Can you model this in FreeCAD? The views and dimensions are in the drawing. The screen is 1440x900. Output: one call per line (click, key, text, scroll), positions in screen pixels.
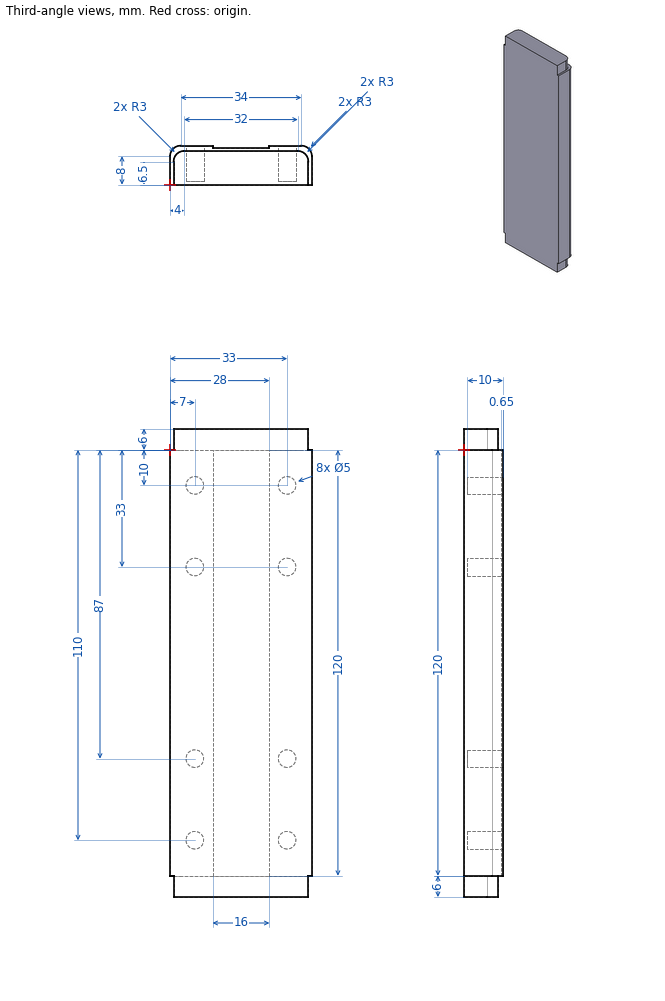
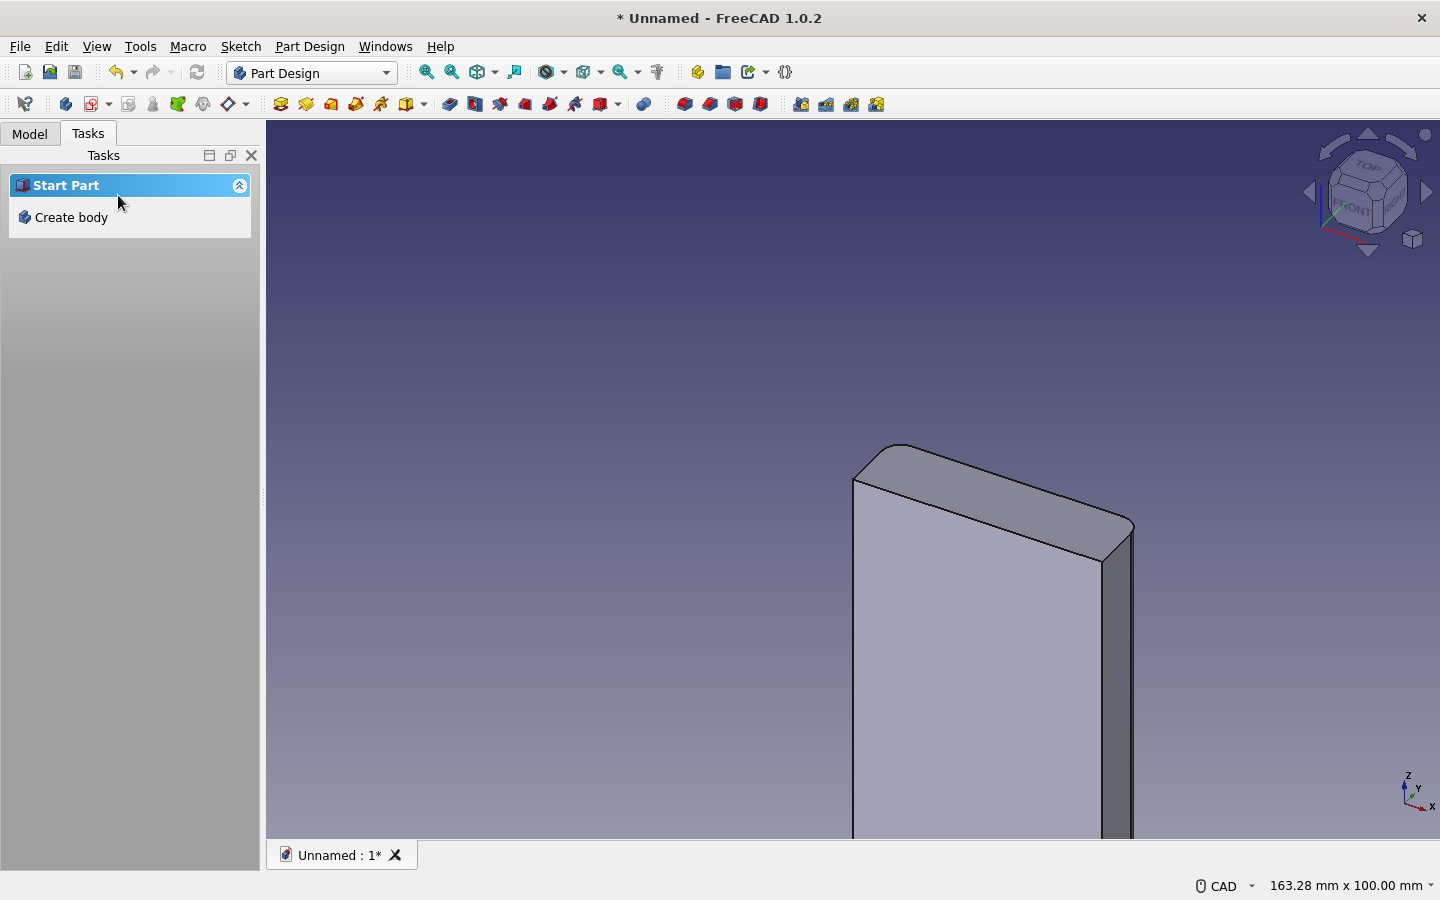
click(427, 72)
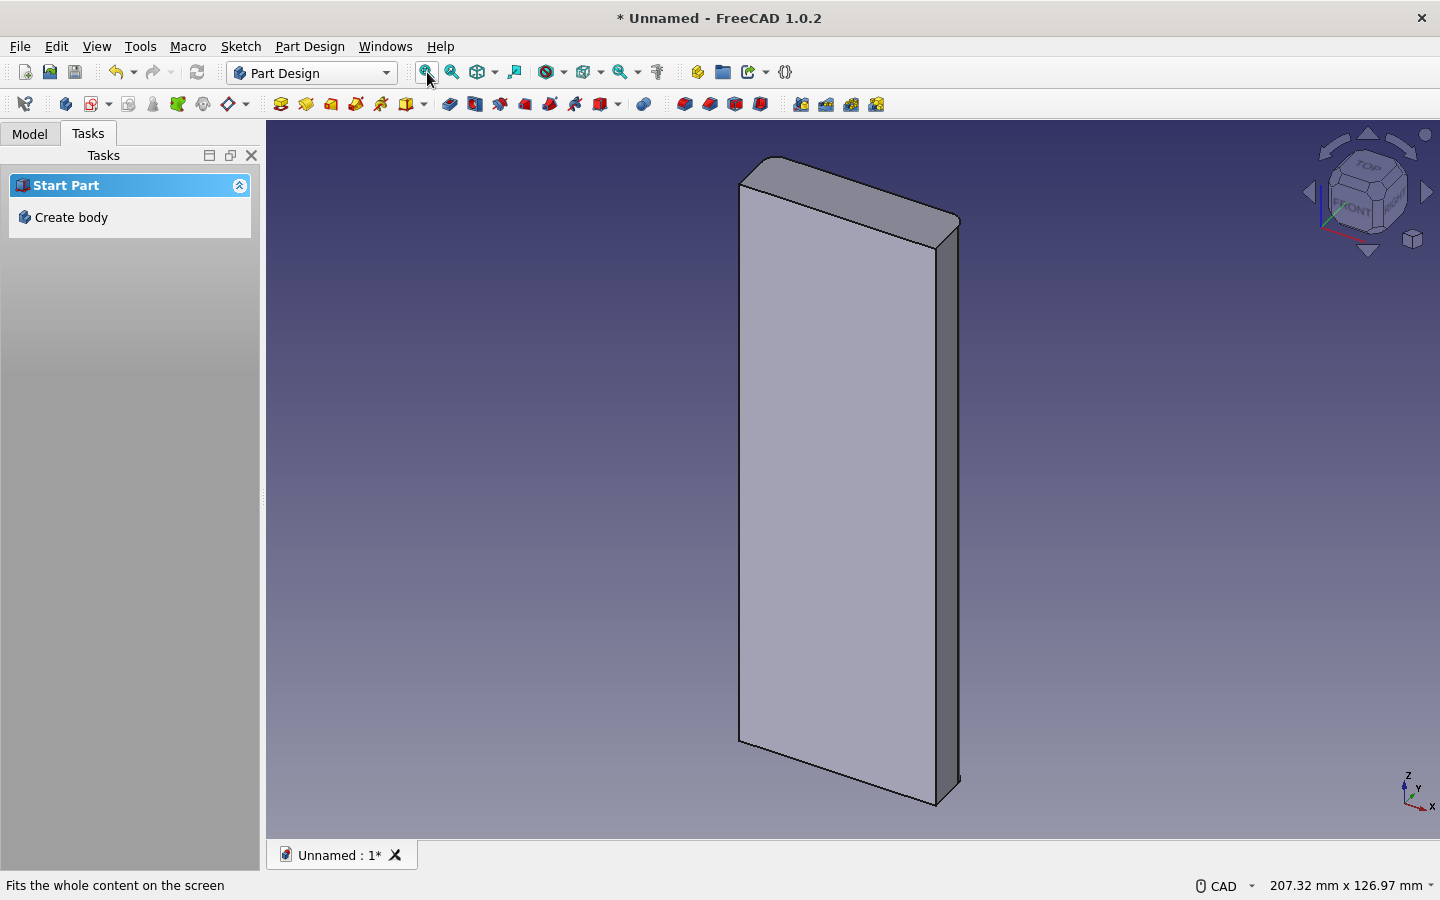
click(90, 104)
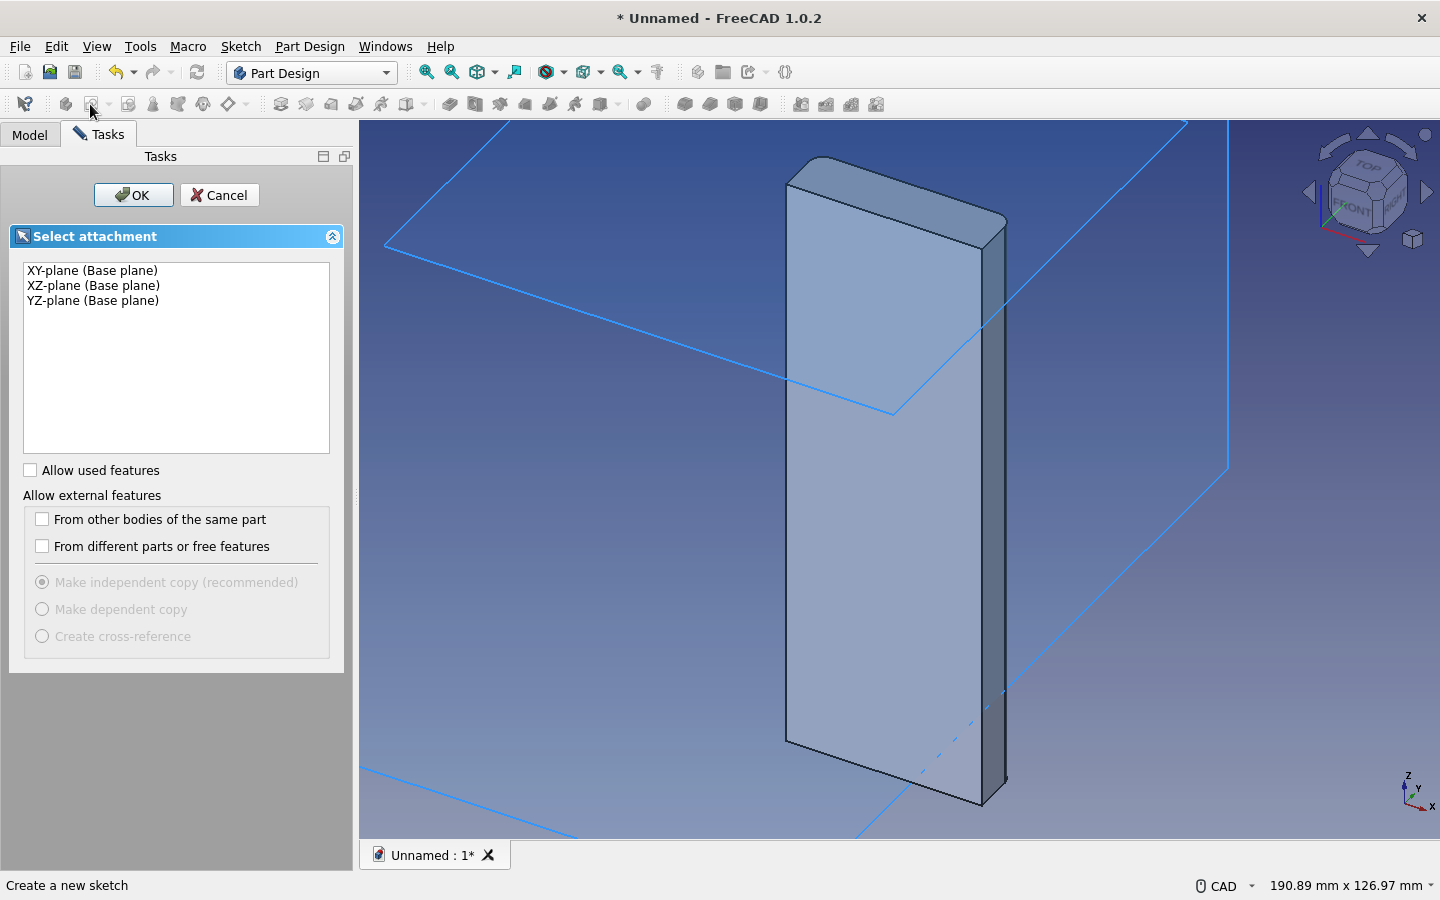
click(84, 270)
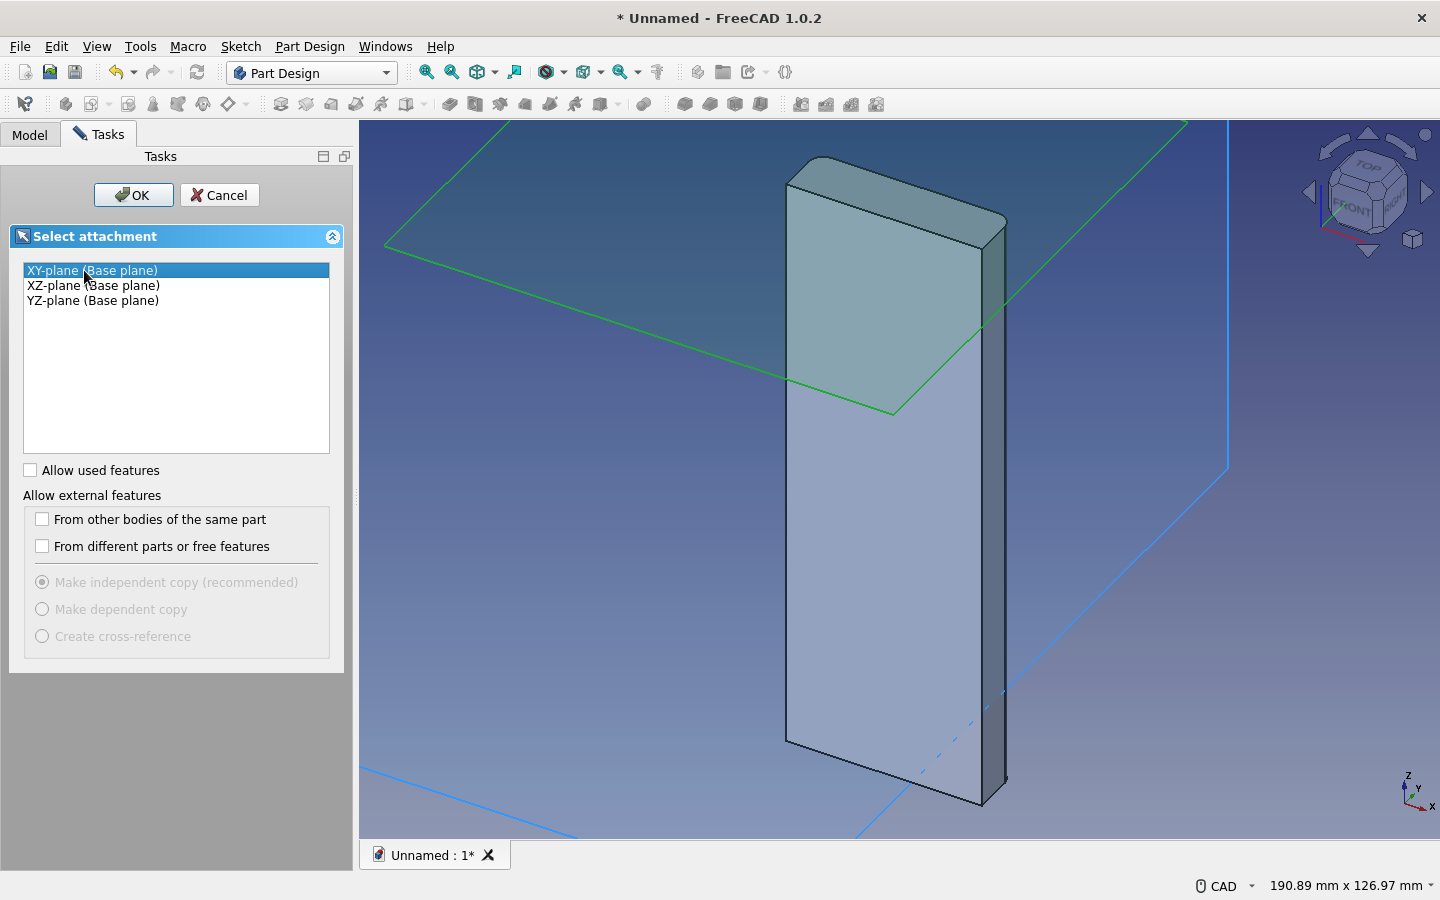
click(134, 195)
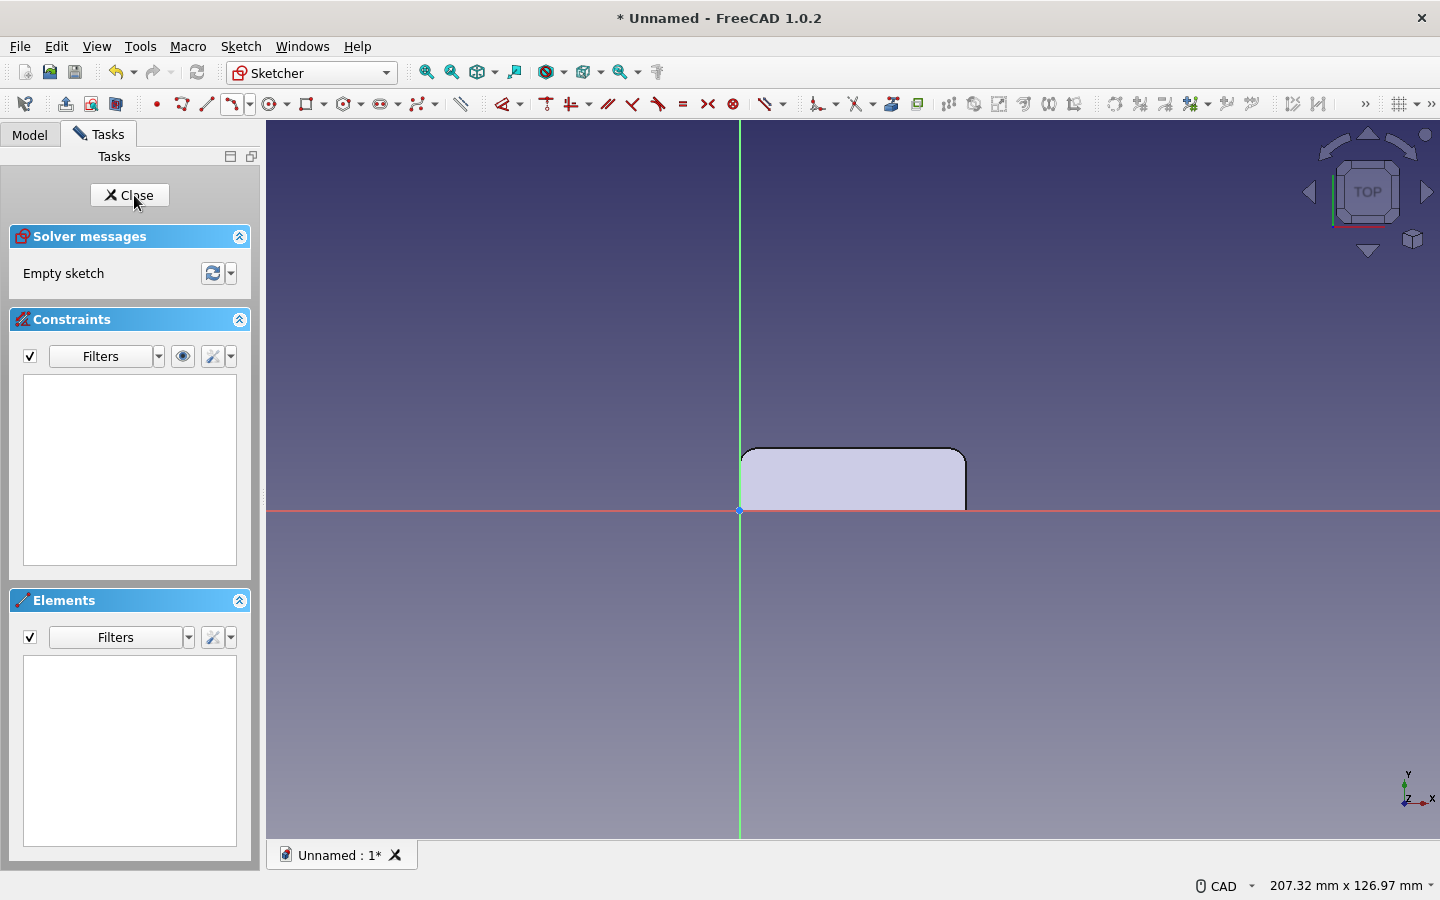
scroll(878, 486, up, 6)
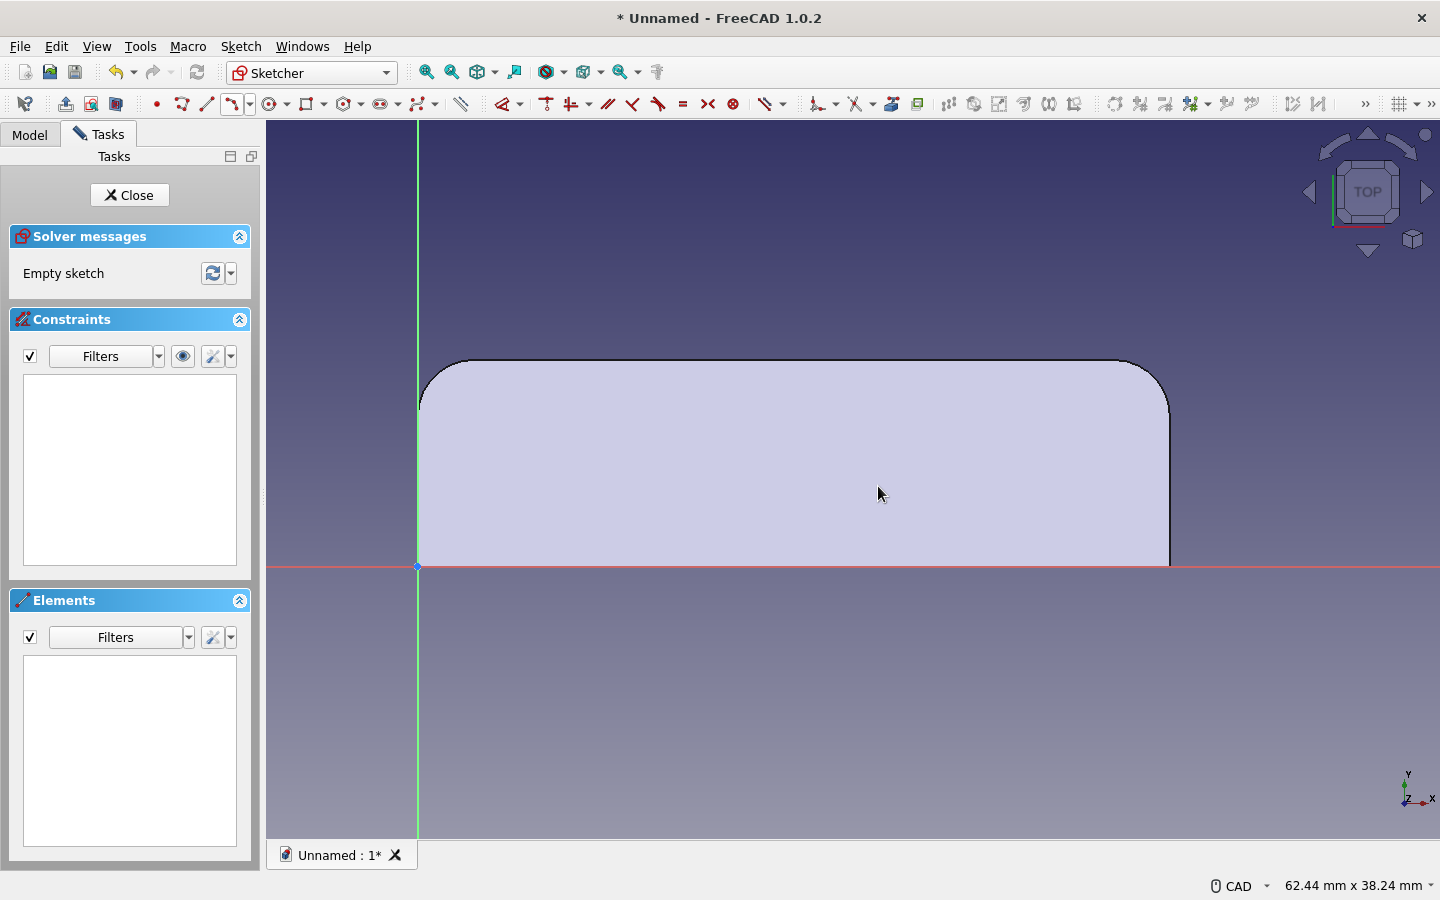
click(207, 104)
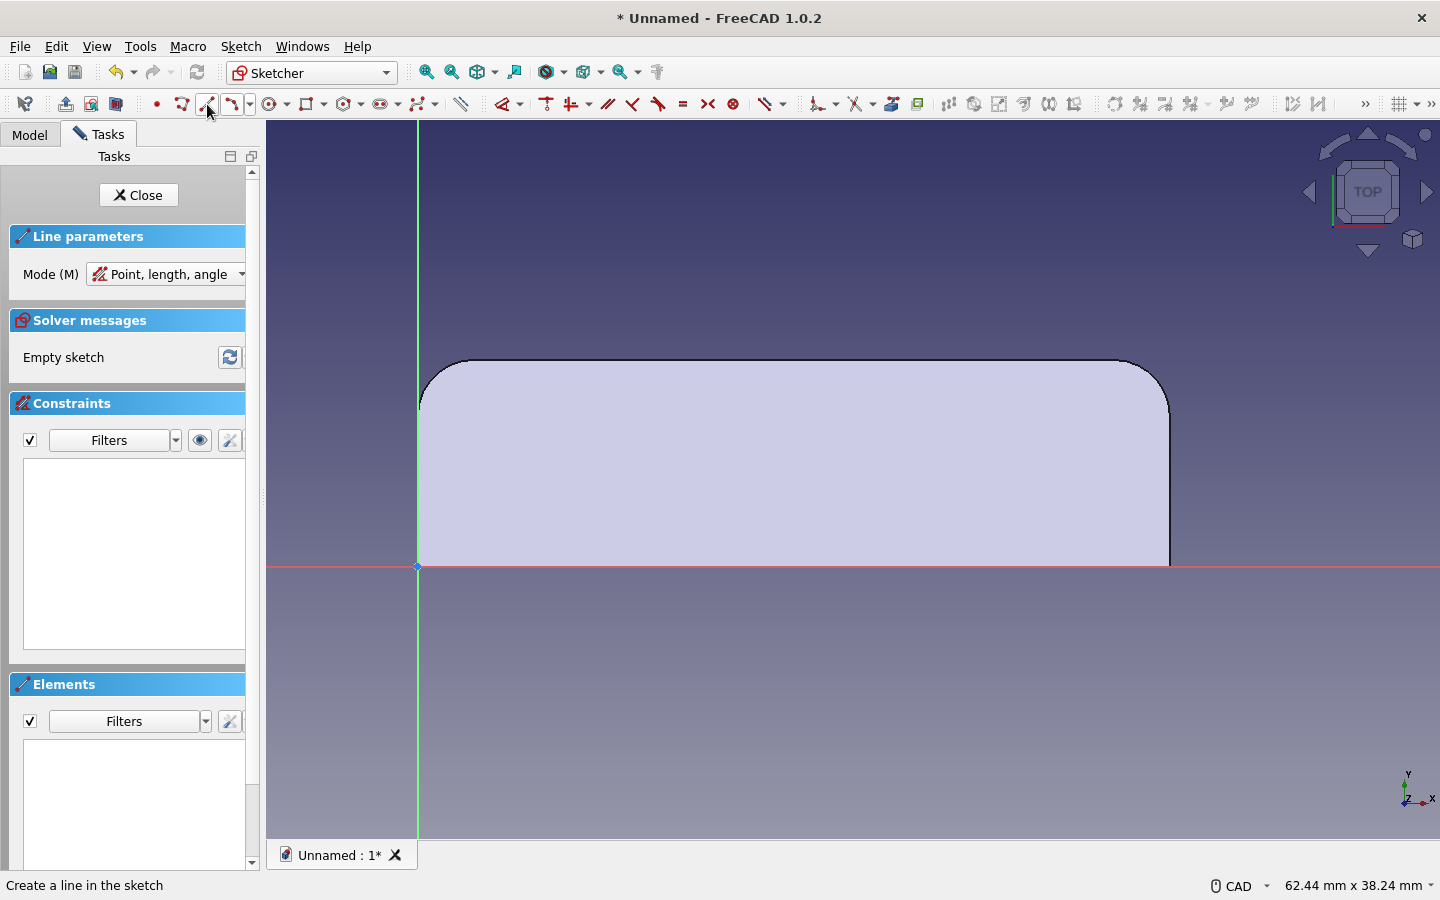
click(1095, 388)
click(493, 388)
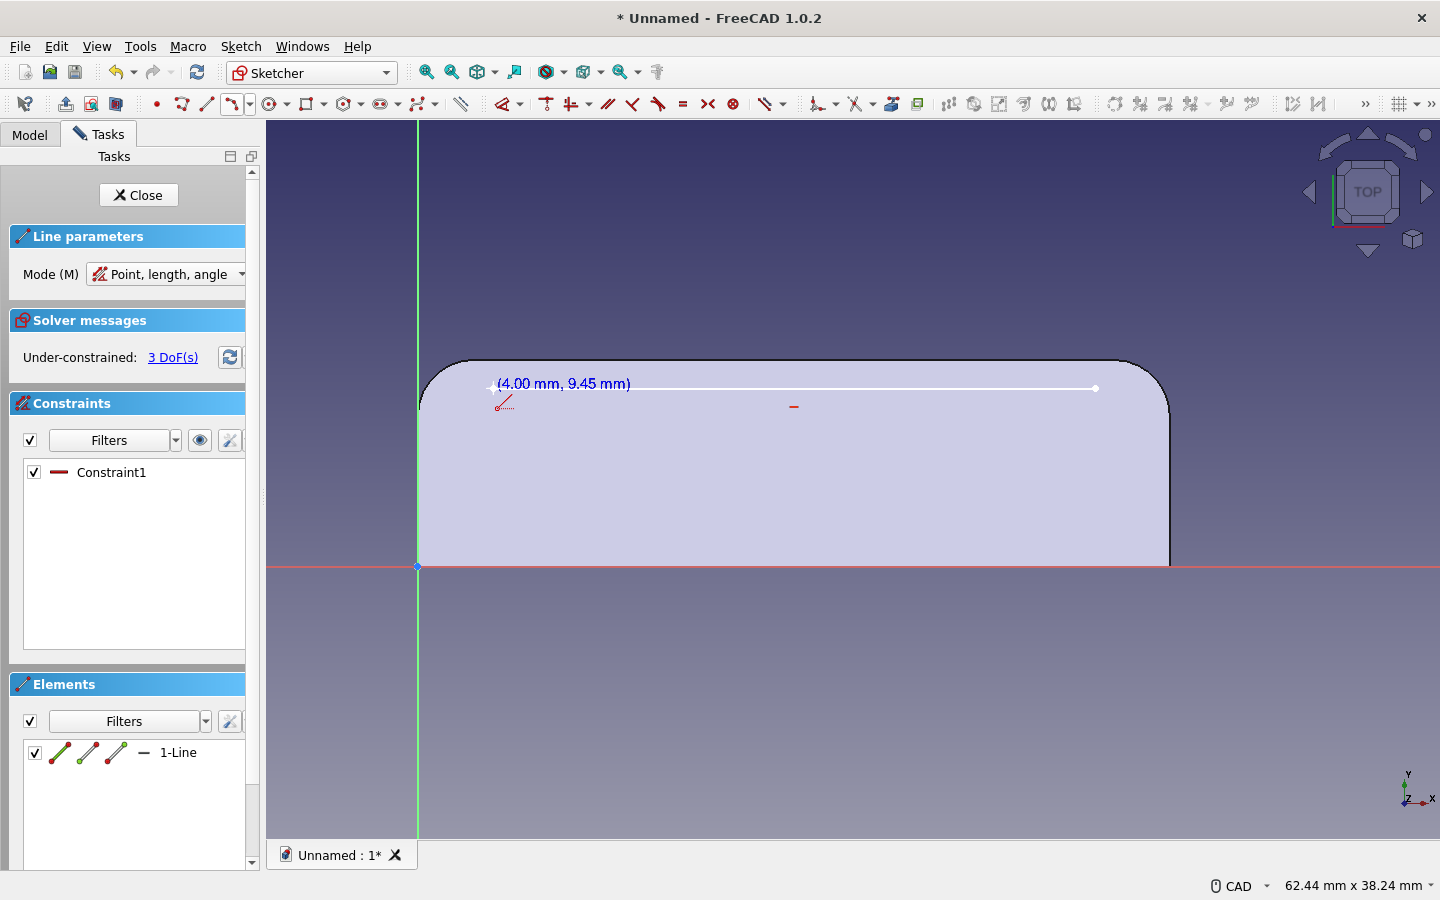
click(182, 104)